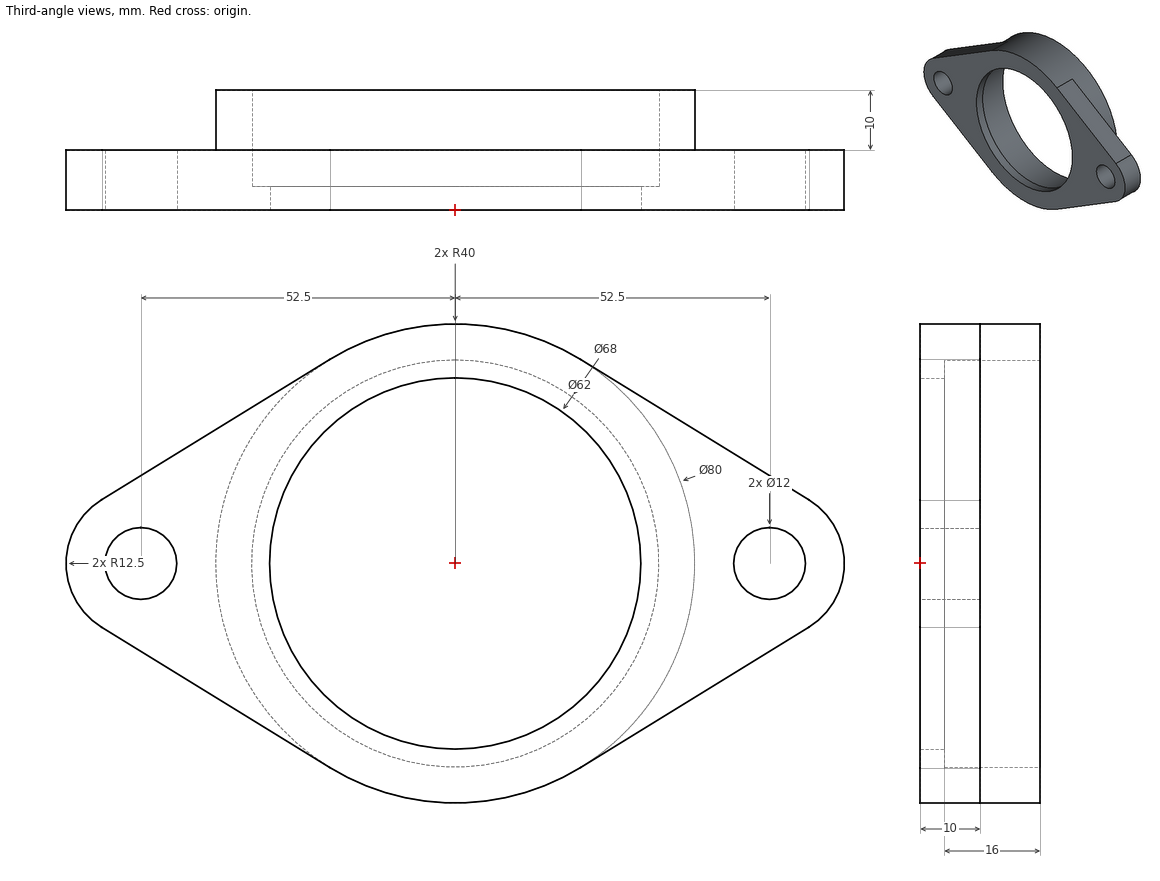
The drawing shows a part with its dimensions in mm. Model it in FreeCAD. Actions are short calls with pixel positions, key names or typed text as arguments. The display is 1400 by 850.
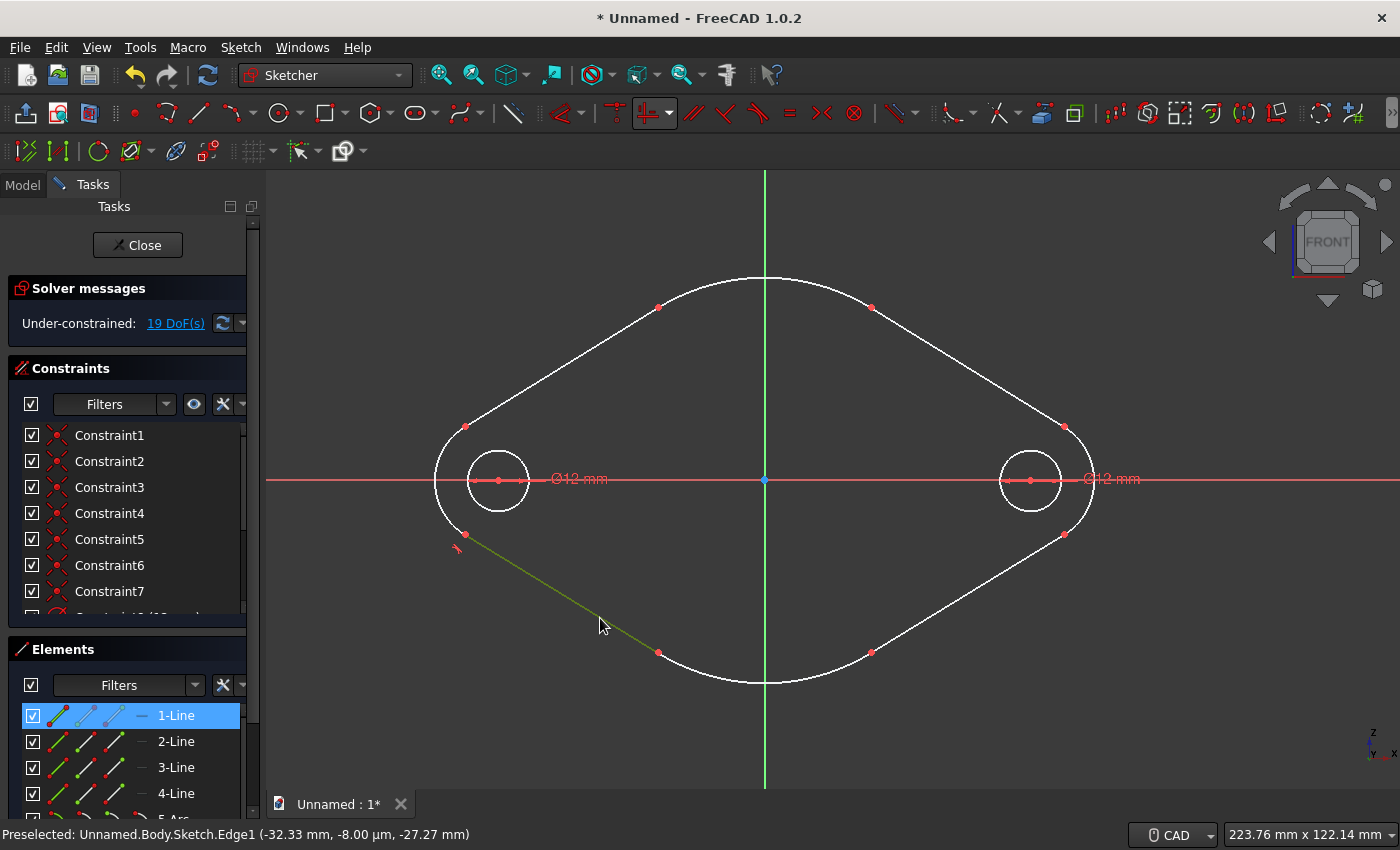
click(720, 678)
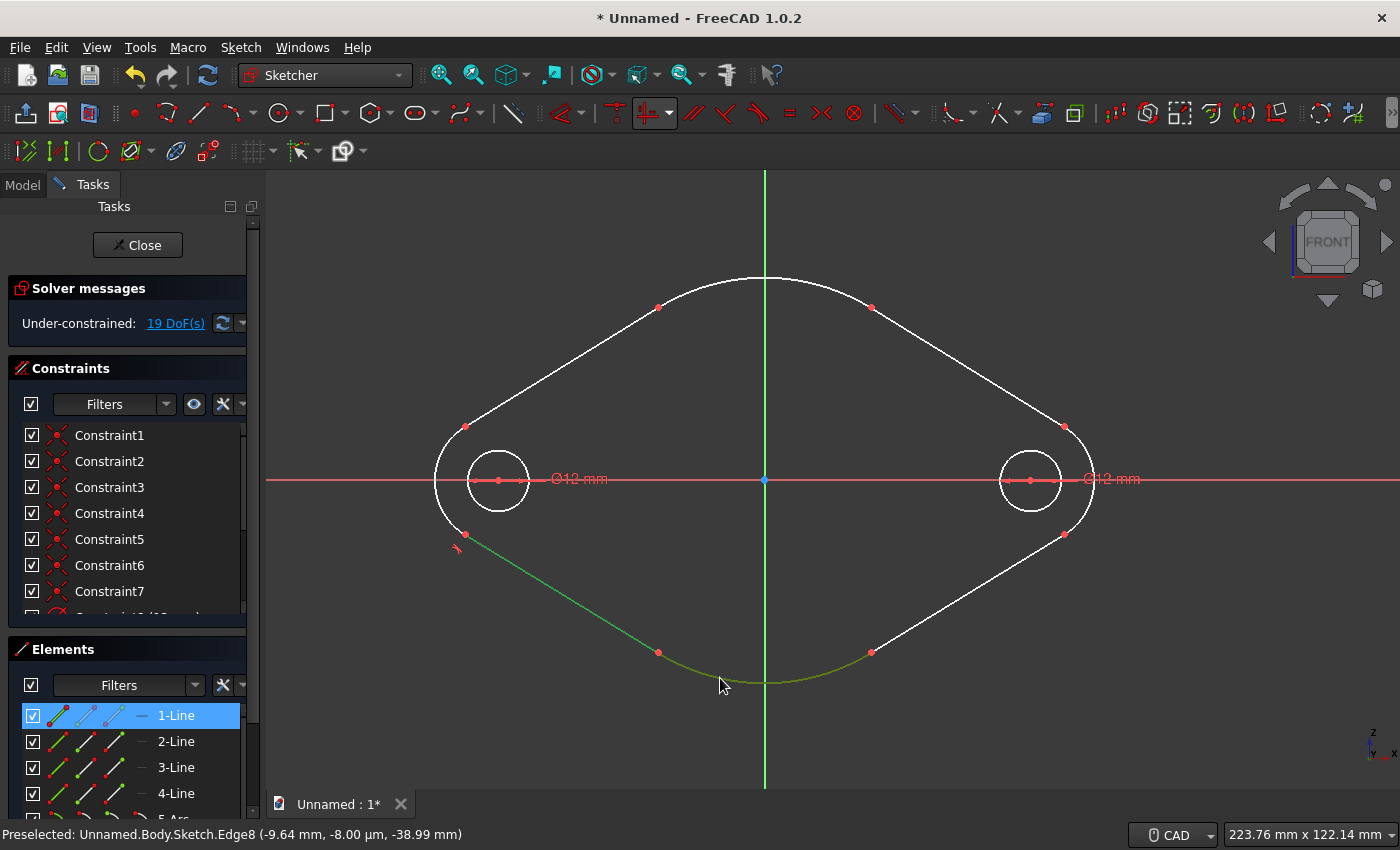
click(758, 114)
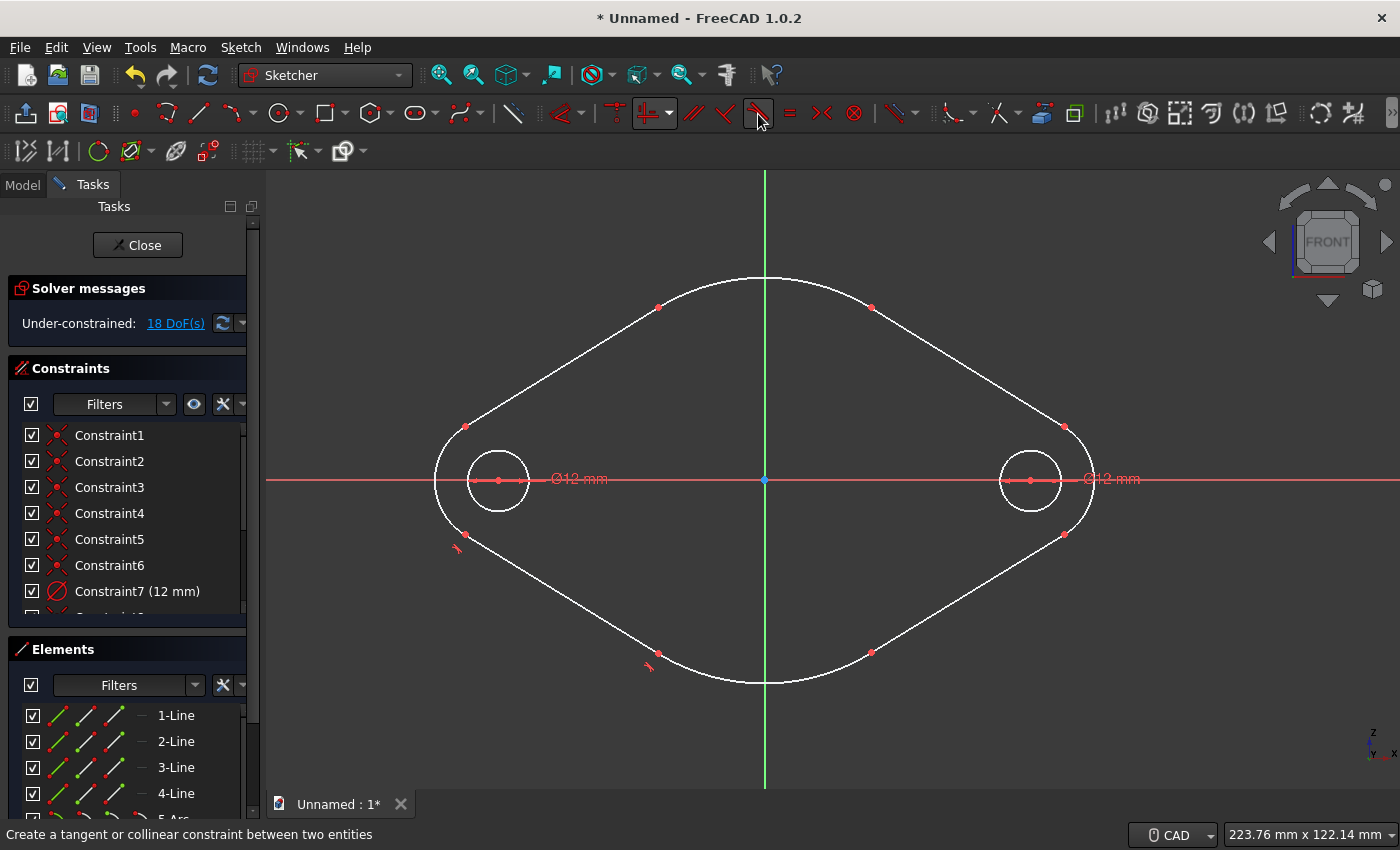
click(523, 391)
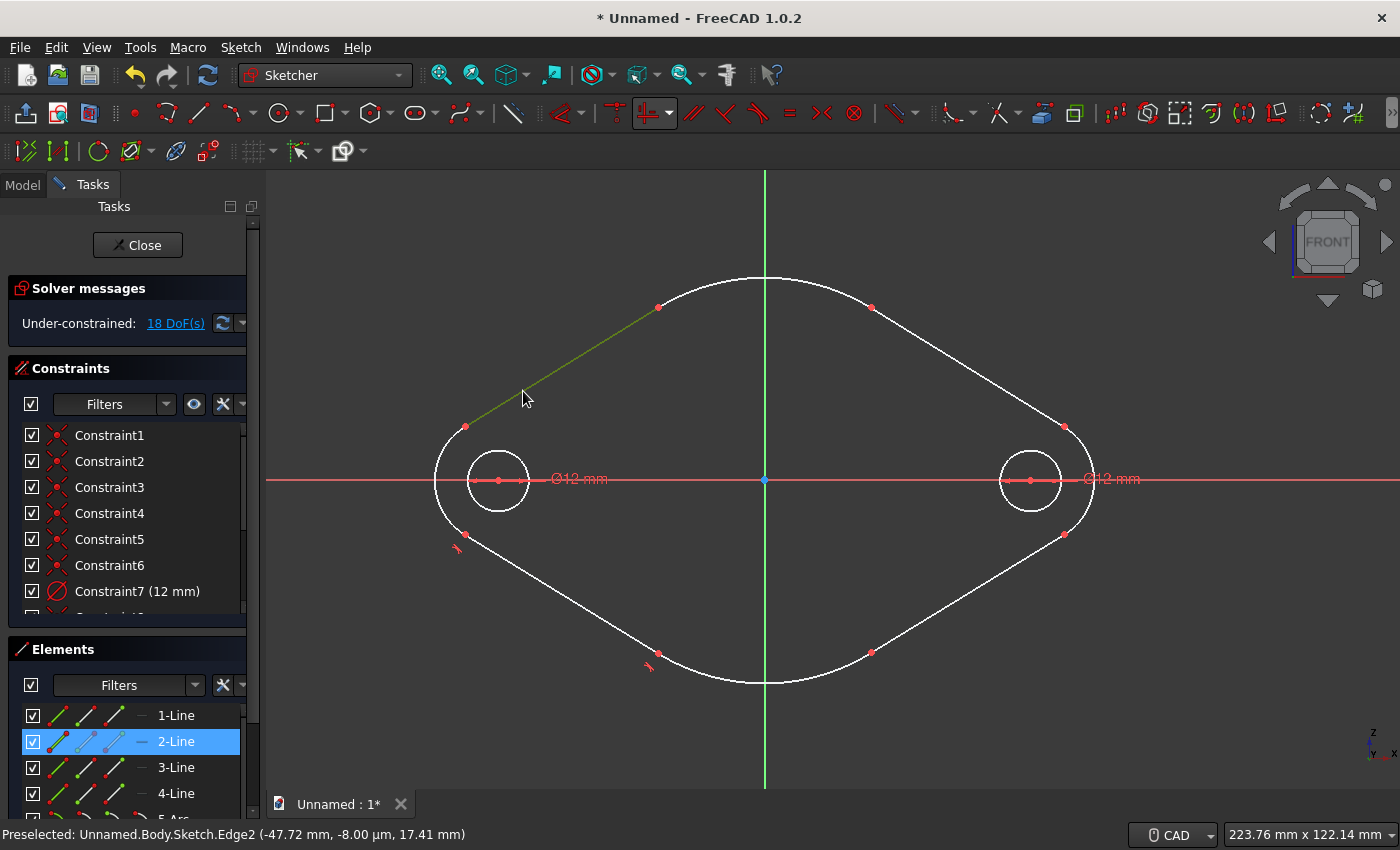
click(440, 456)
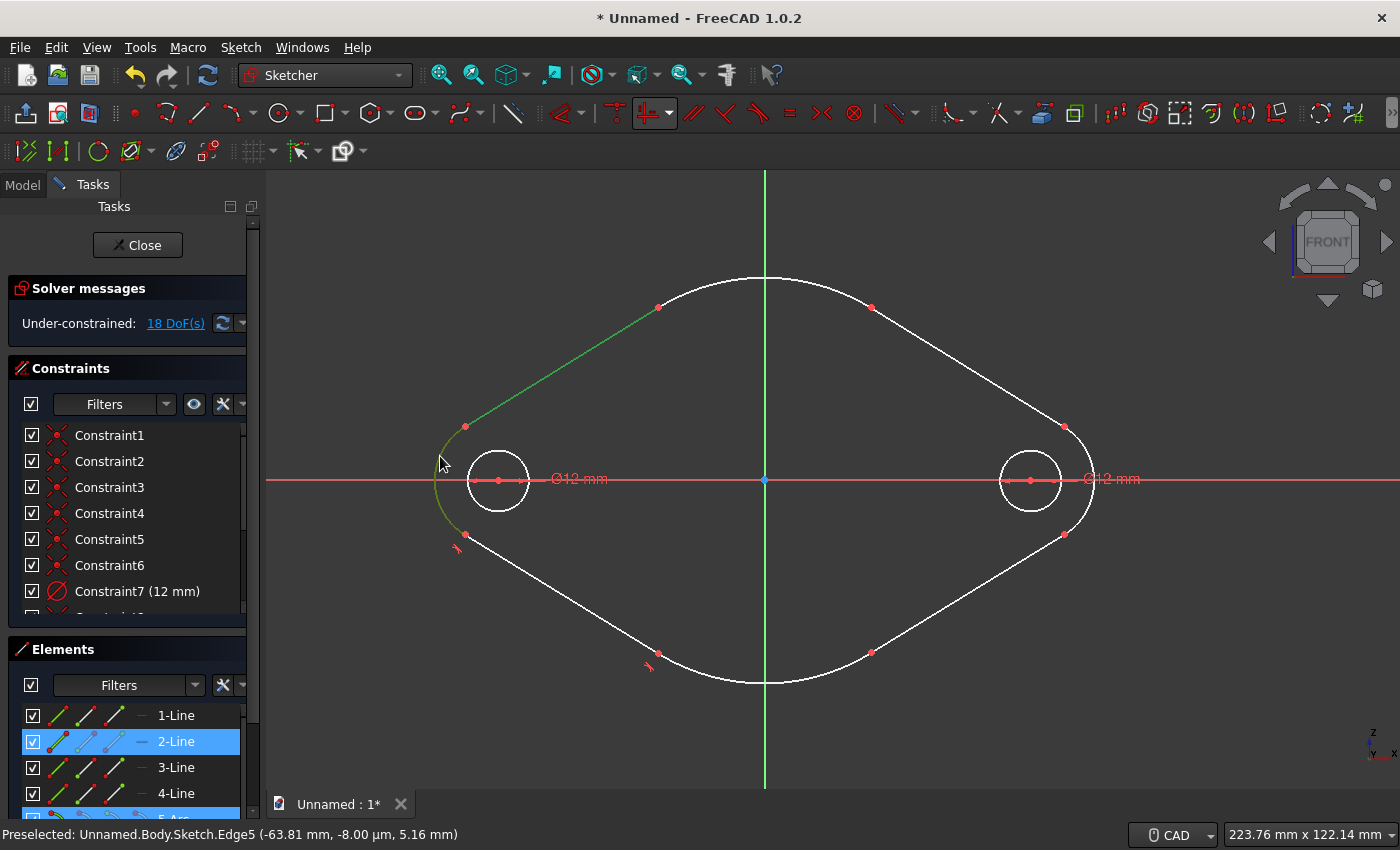
click(758, 114)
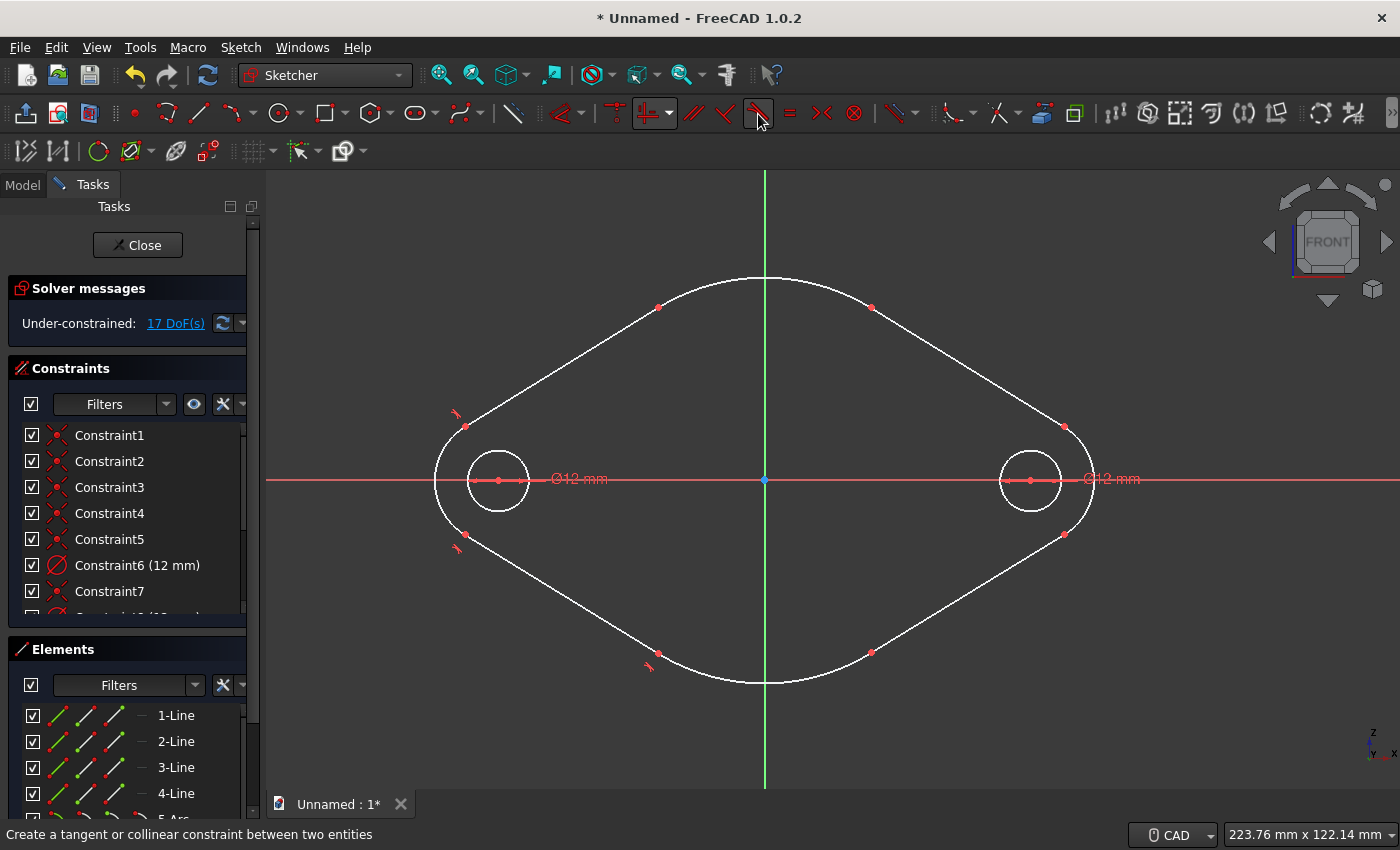
click(523, 391)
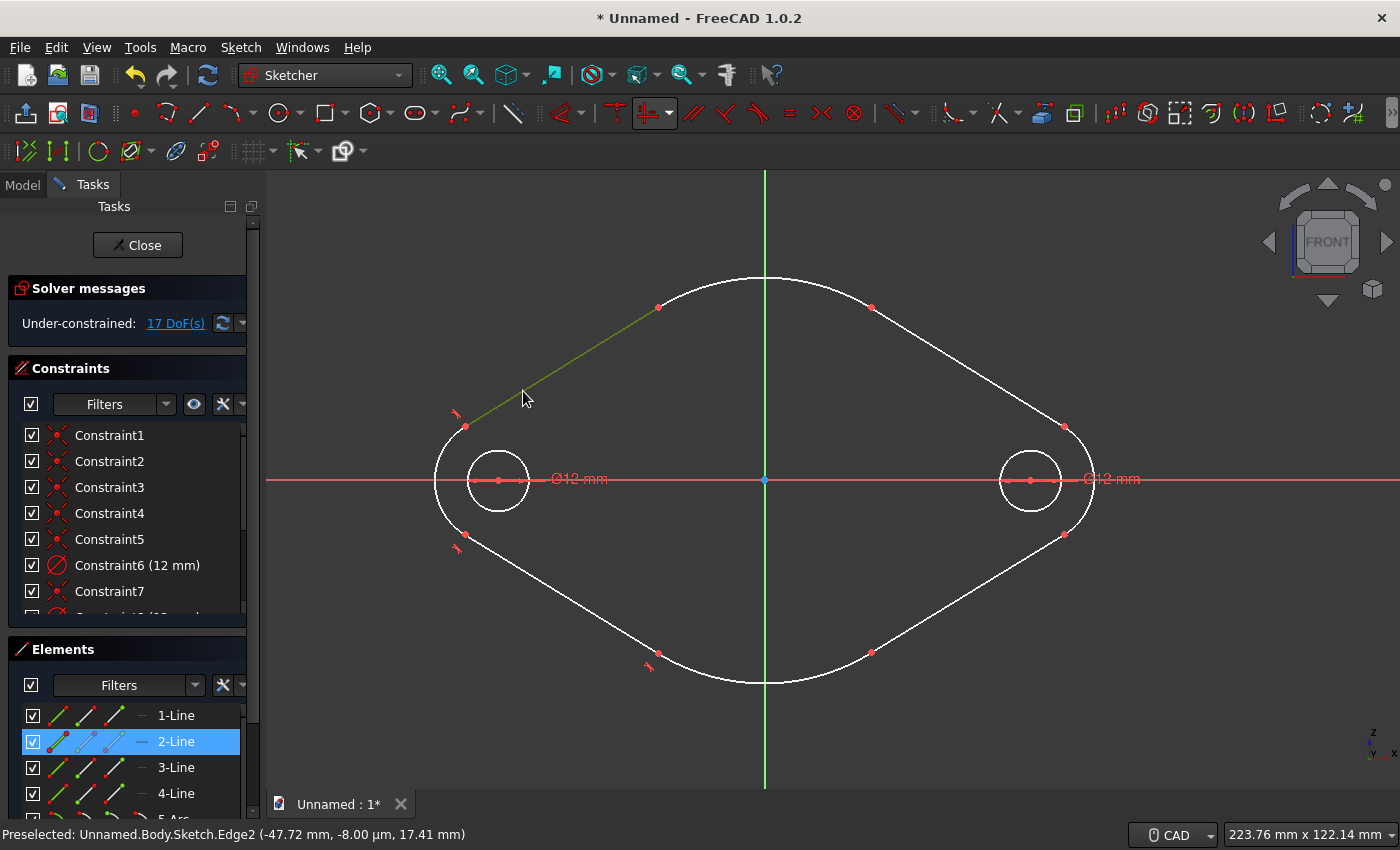
click(809, 283)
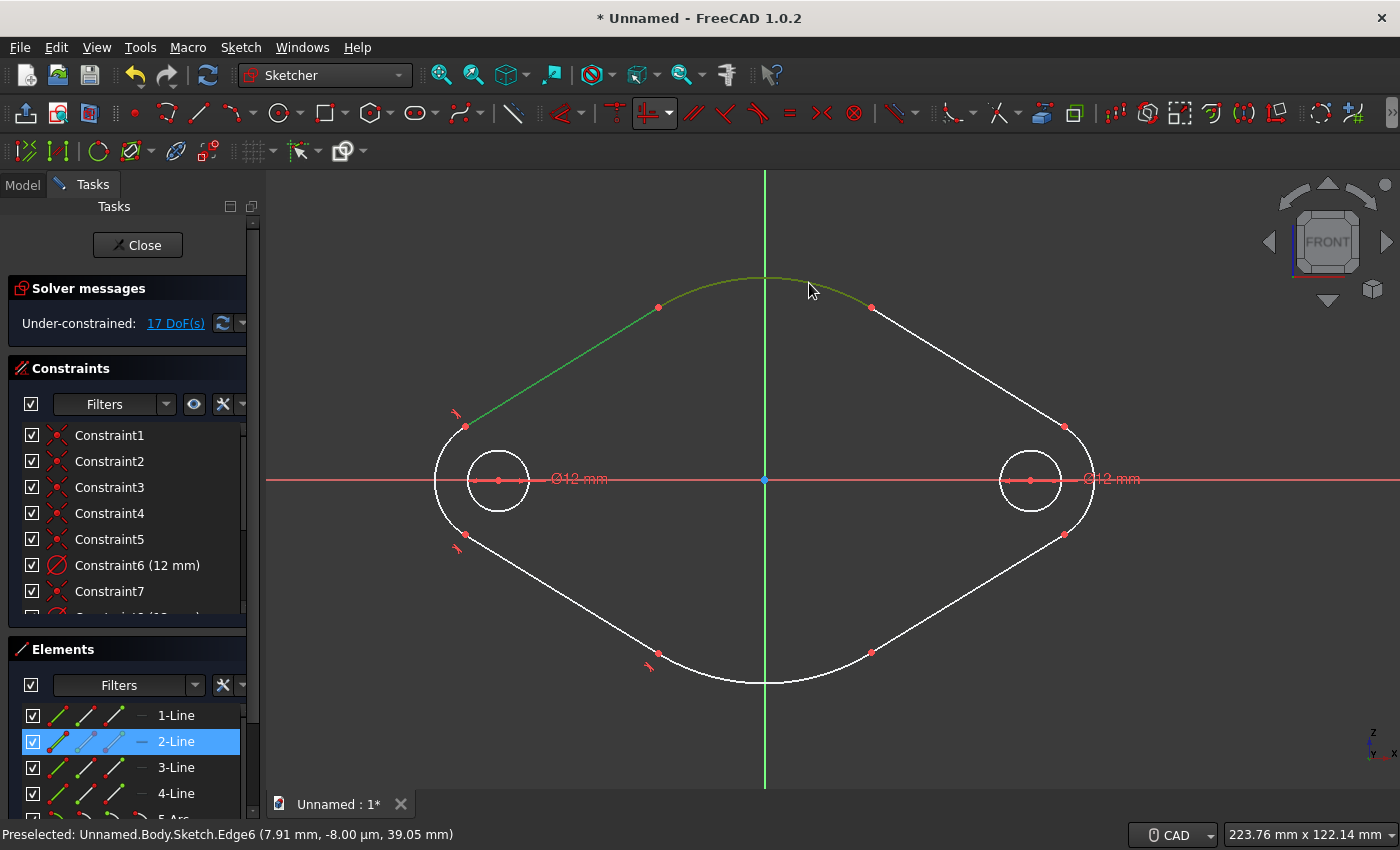
click(758, 114)